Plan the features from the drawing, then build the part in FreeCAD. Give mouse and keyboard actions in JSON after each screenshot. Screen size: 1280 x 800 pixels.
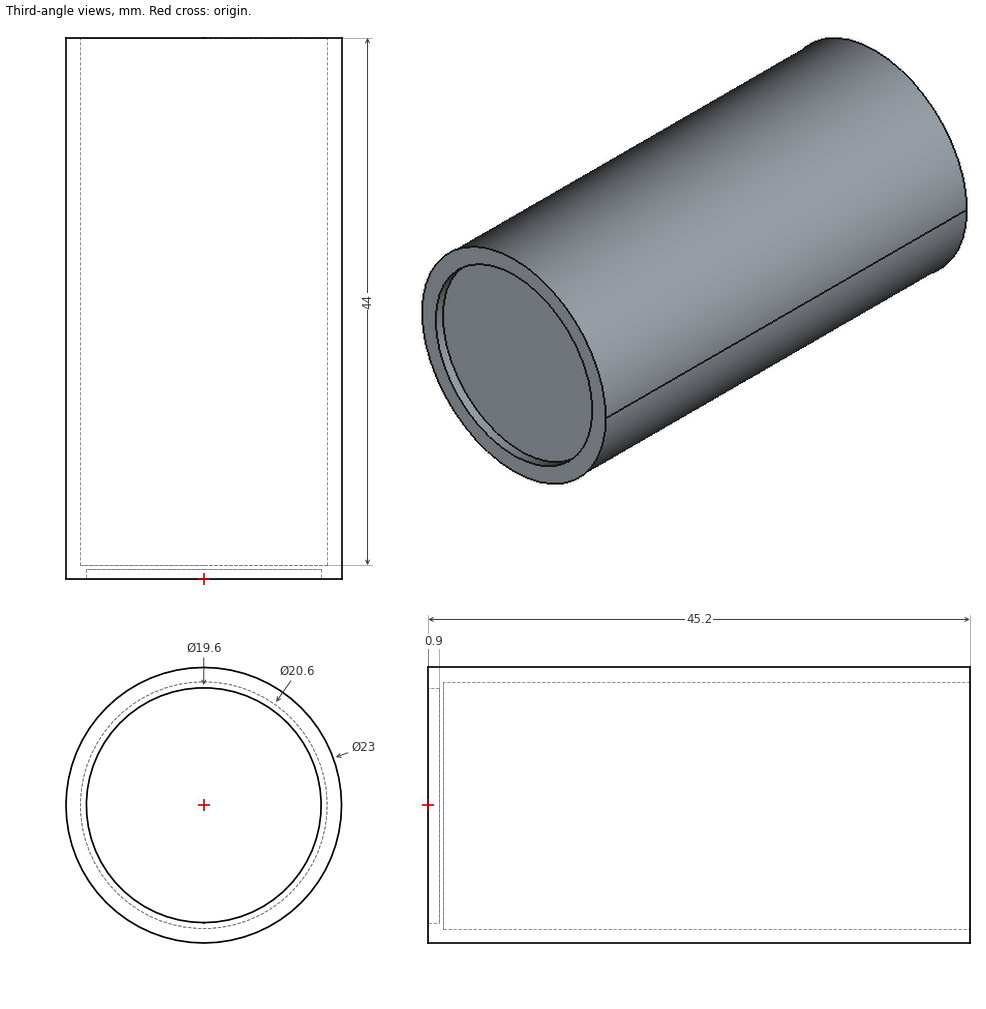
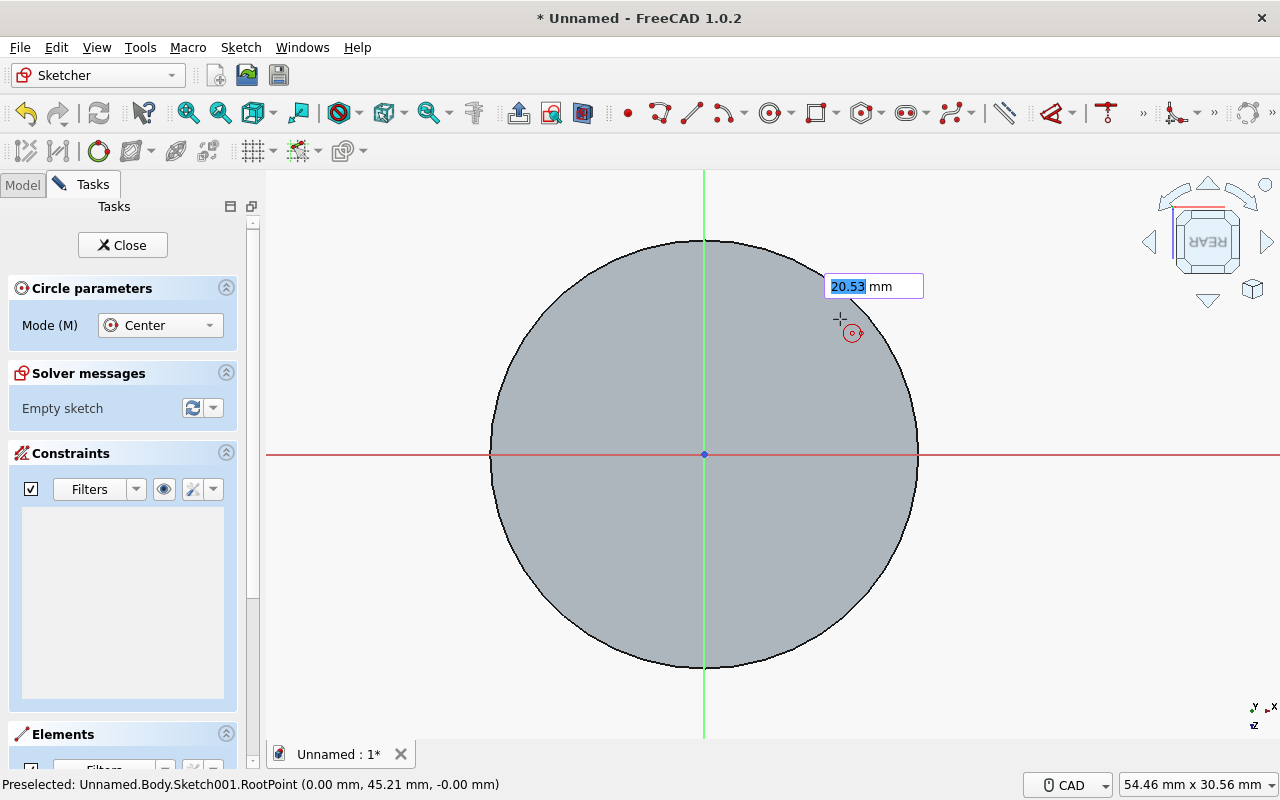
{"action": "type", "text": "20.6"}
{"action": "key", "text": "Return"}
{"action": "key", "text": "Escape"}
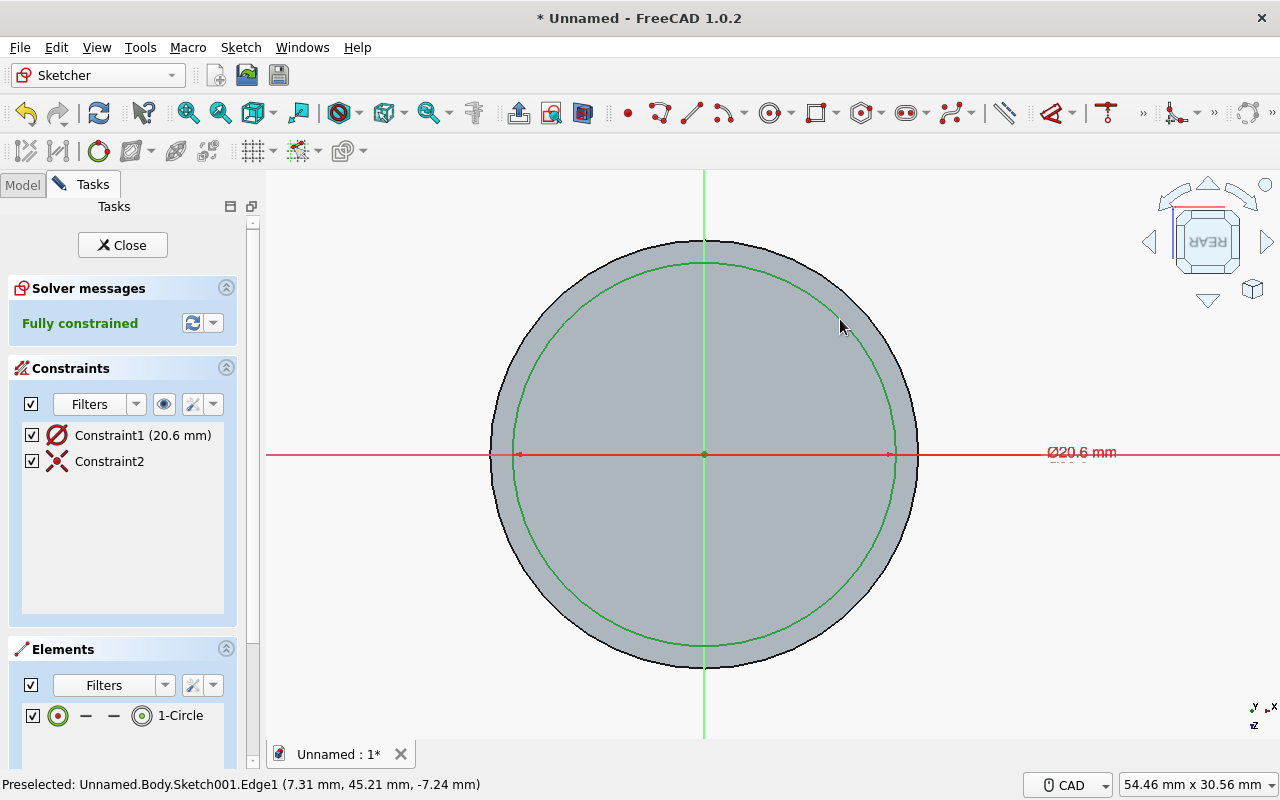
{"action": "left_click", "coordinate": [123, 245]}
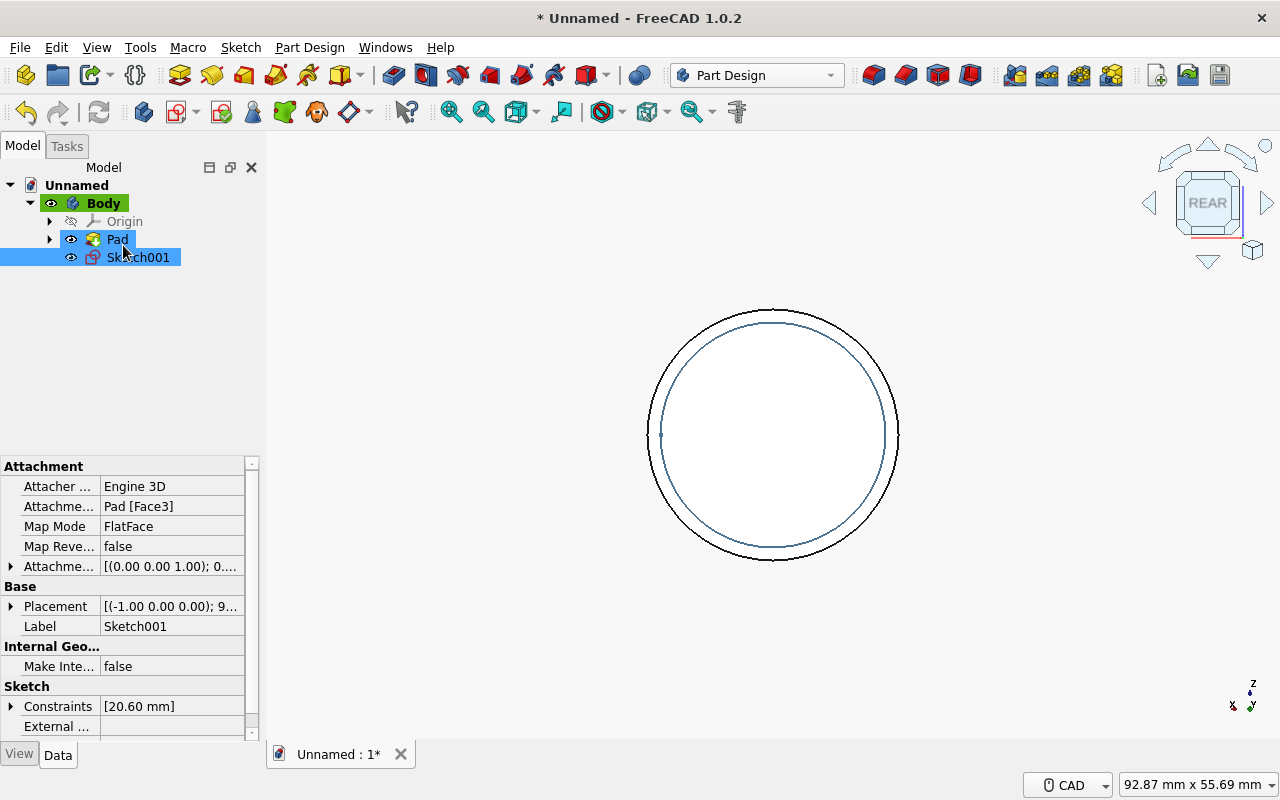
{"action": "left_click", "coordinate": [394, 76]}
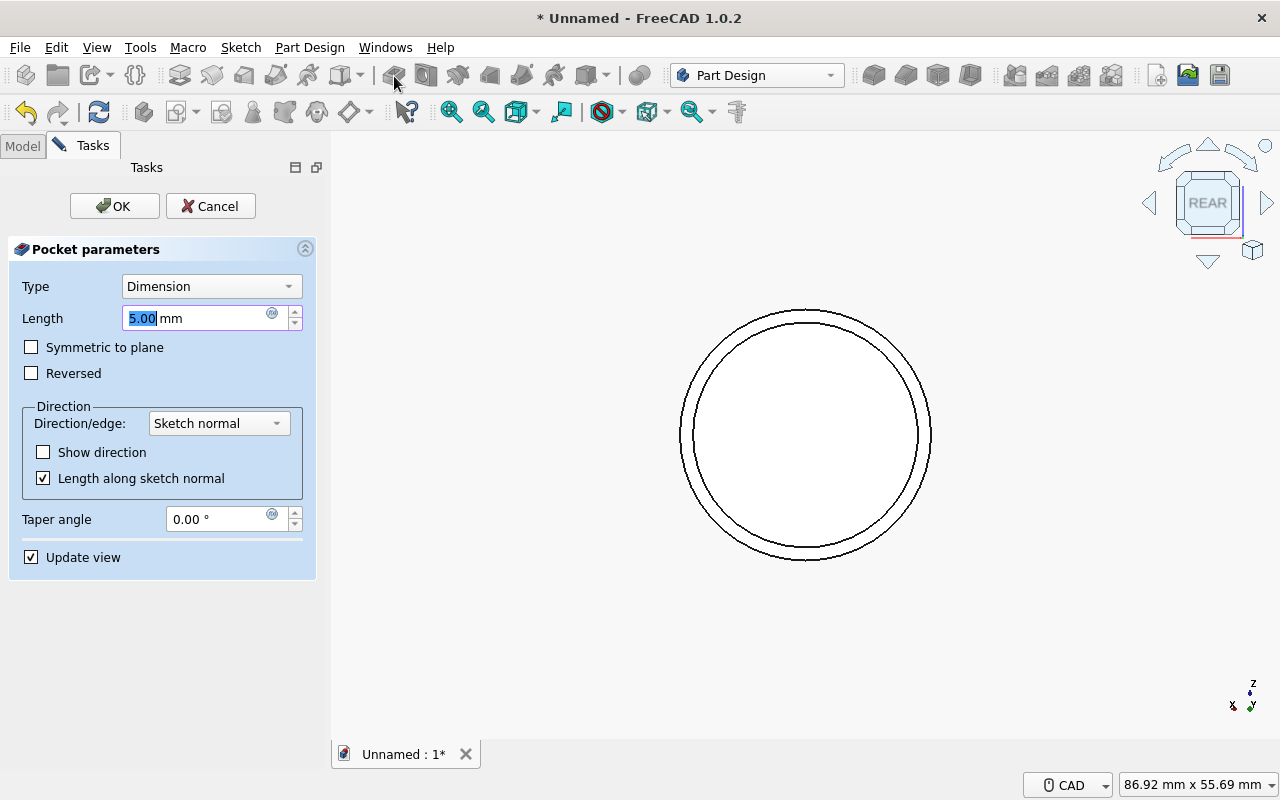
{"action": "type", "text": "44"}
{"action": "key", "text": "Tab"}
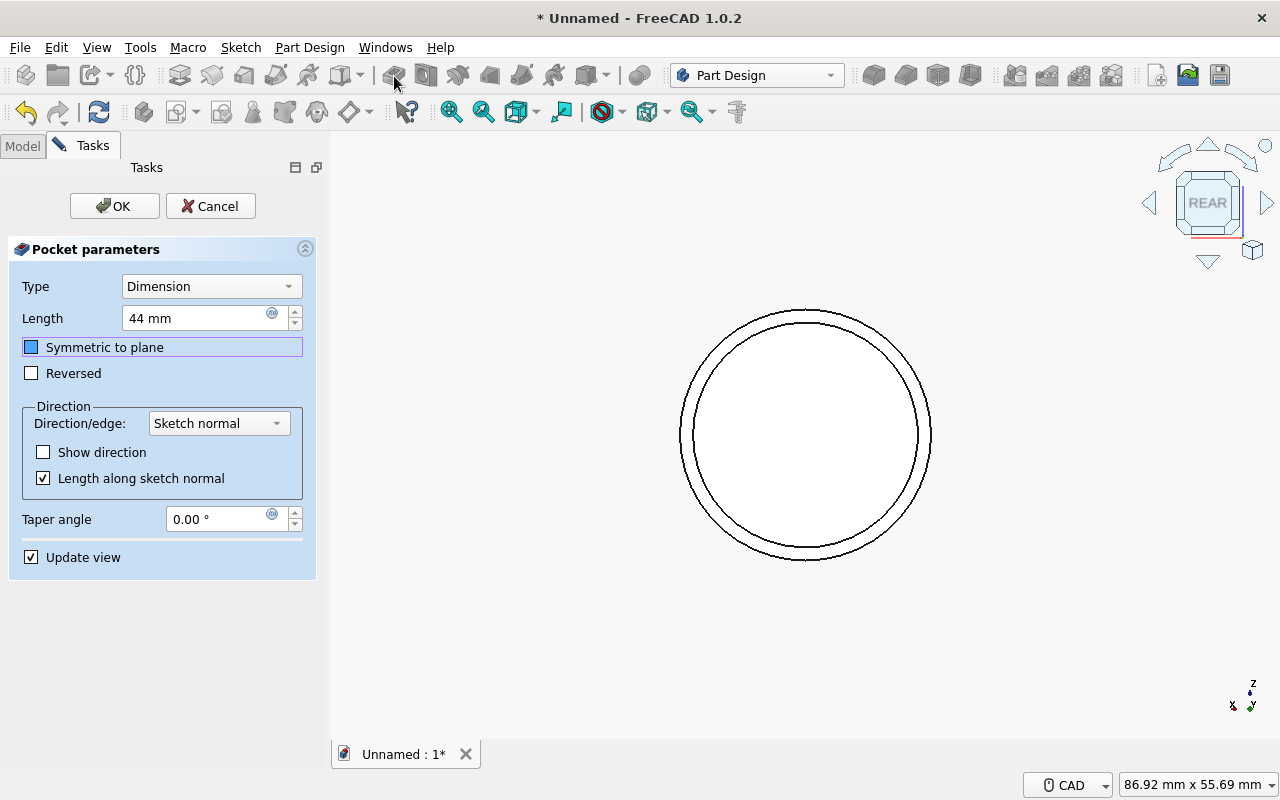
{"action": "left_click", "coordinate": [115, 206]}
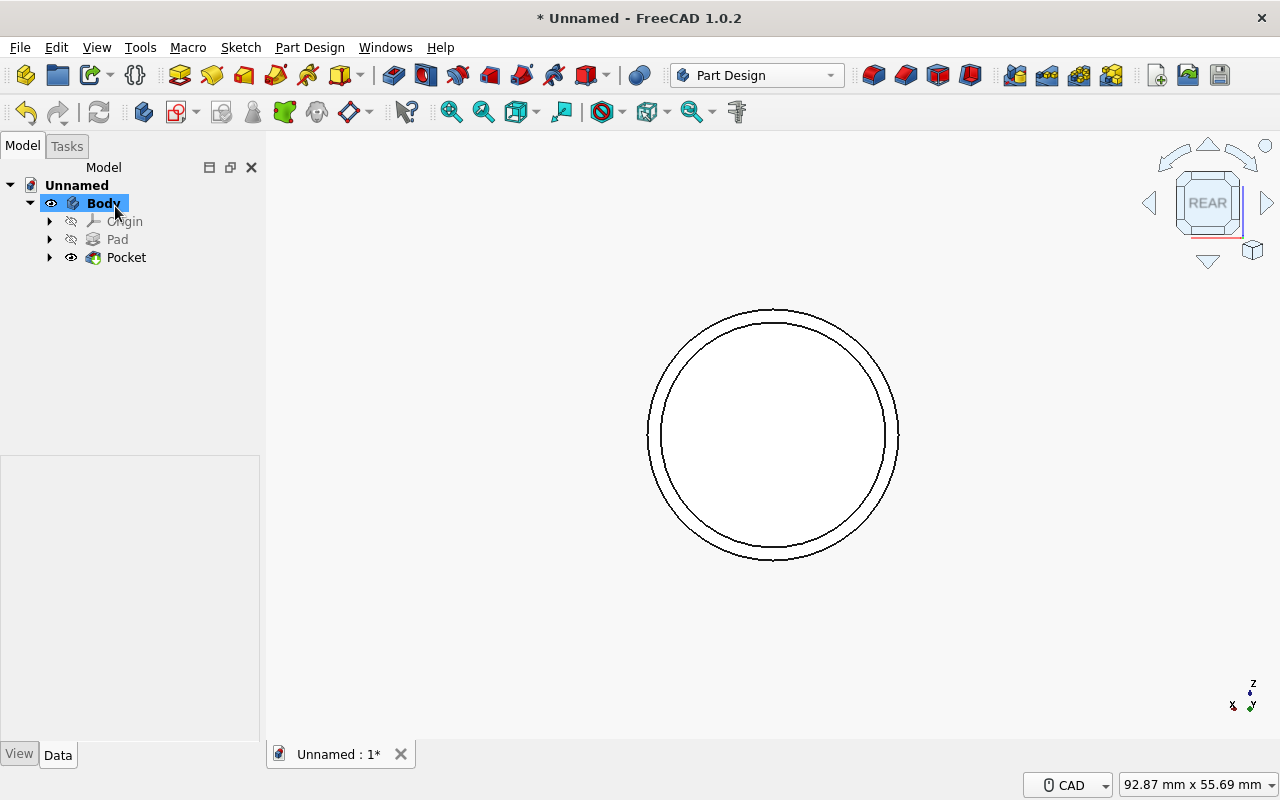
{"action": "left_click", "coordinate": [452, 112]}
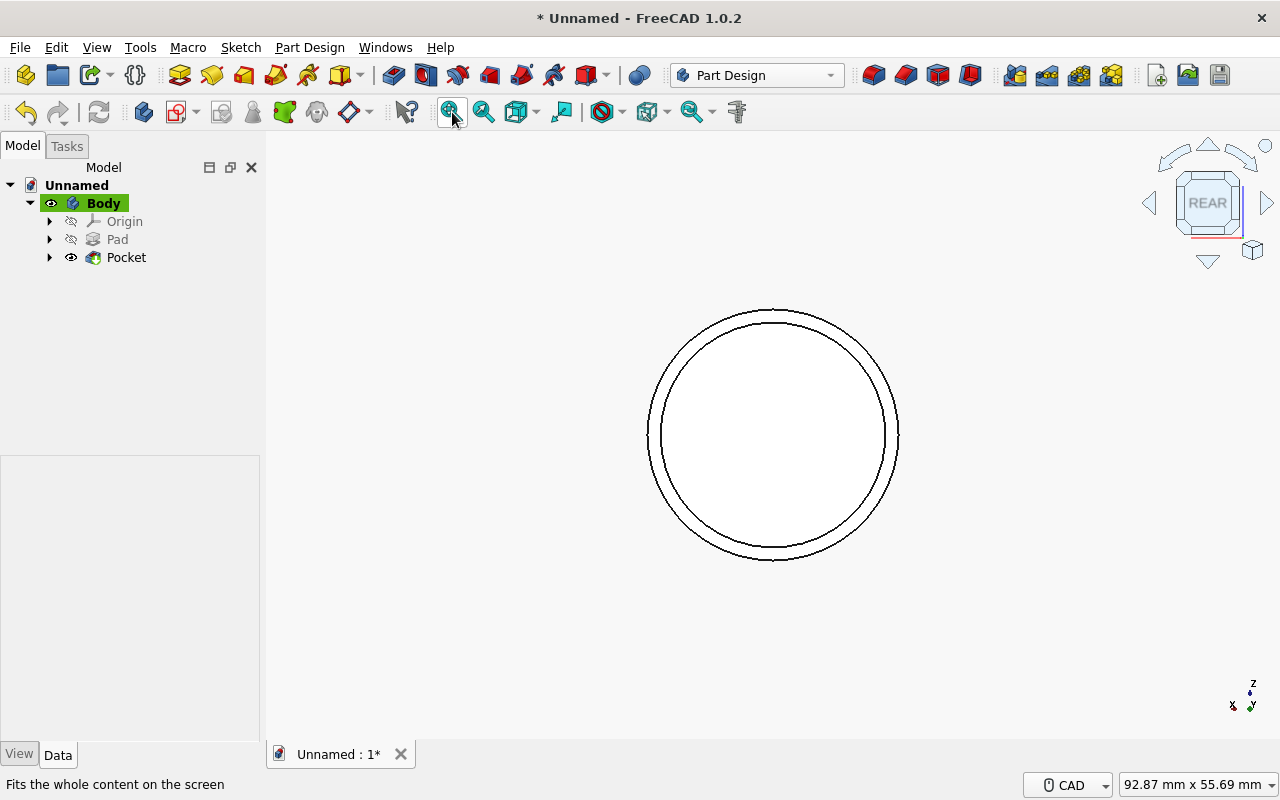
{"action": "key", "text": "0"}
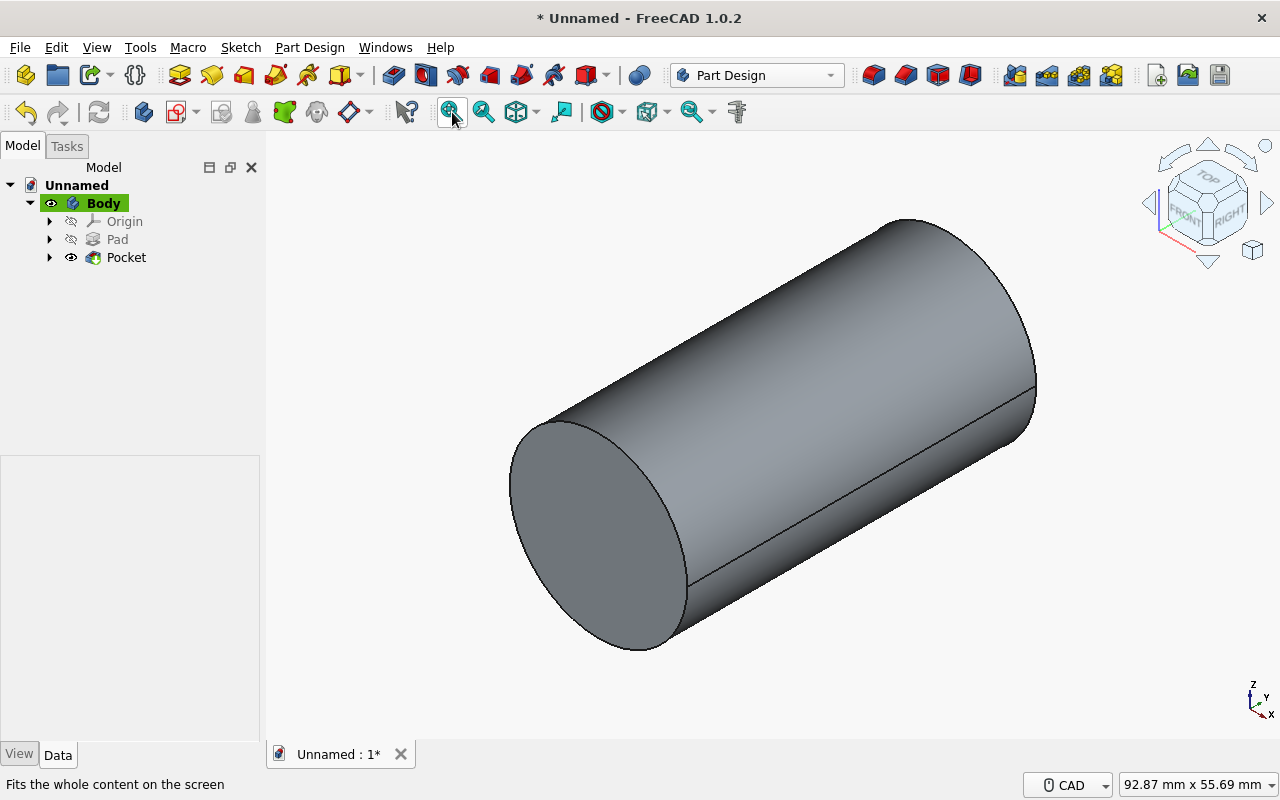
{"action": "left_click", "coordinate": [599, 535]}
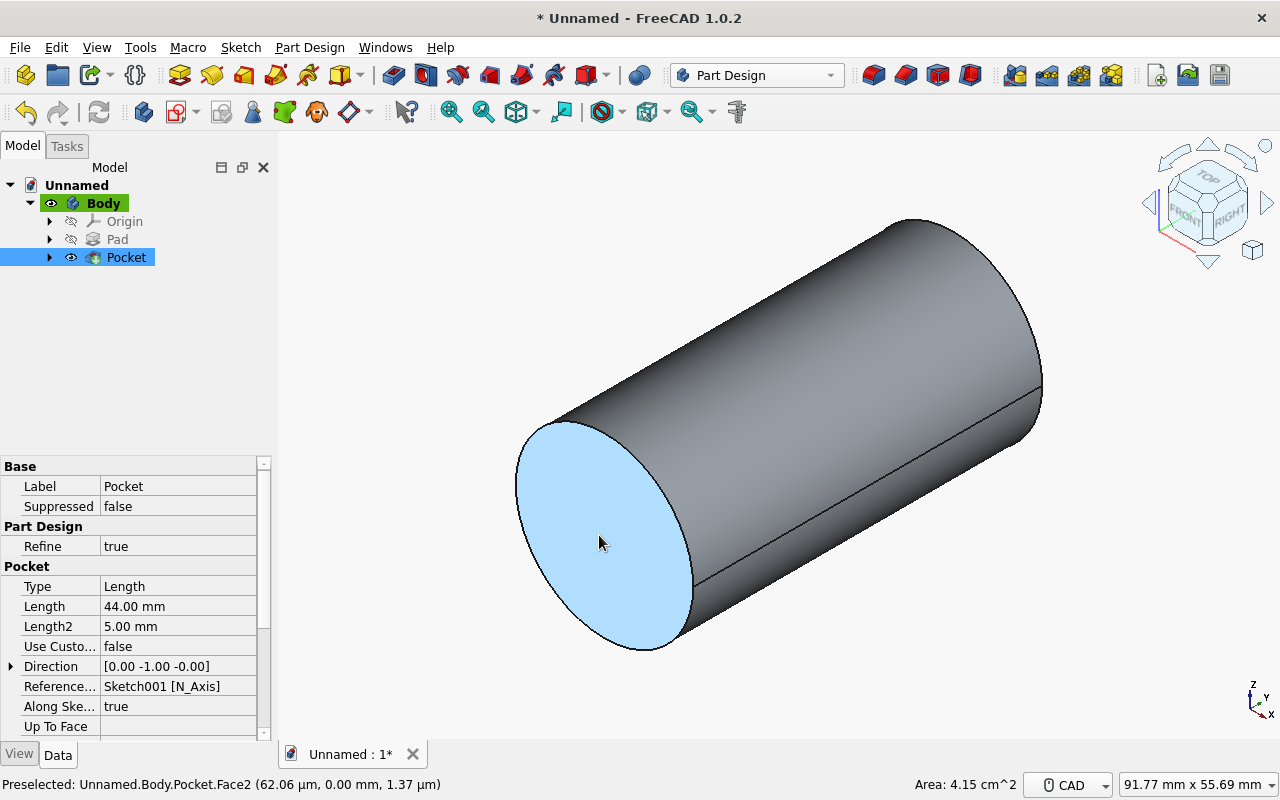
{"action": "left_click", "coordinate": [176, 112]}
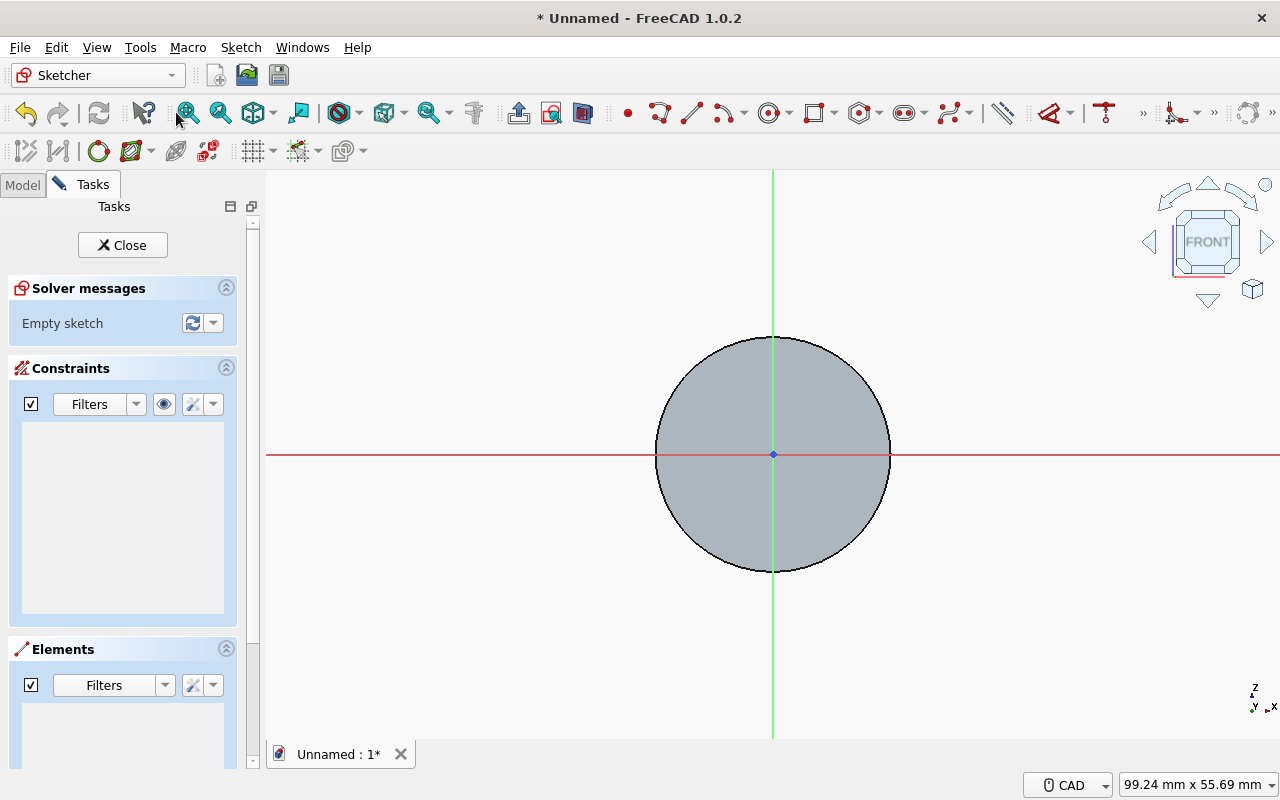
{"action": "scroll", "coordinate": [856, 455], "scroll_direction": "up", "scroll_amount": 3}